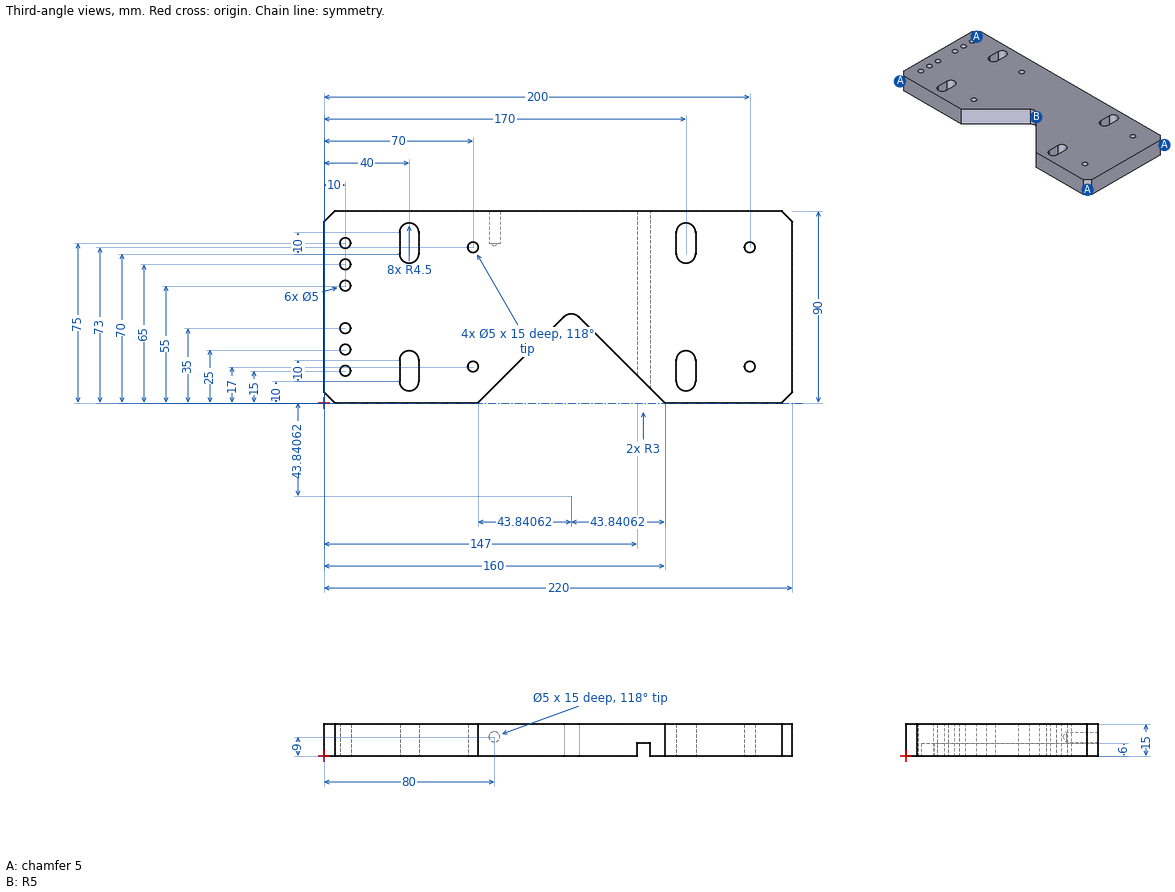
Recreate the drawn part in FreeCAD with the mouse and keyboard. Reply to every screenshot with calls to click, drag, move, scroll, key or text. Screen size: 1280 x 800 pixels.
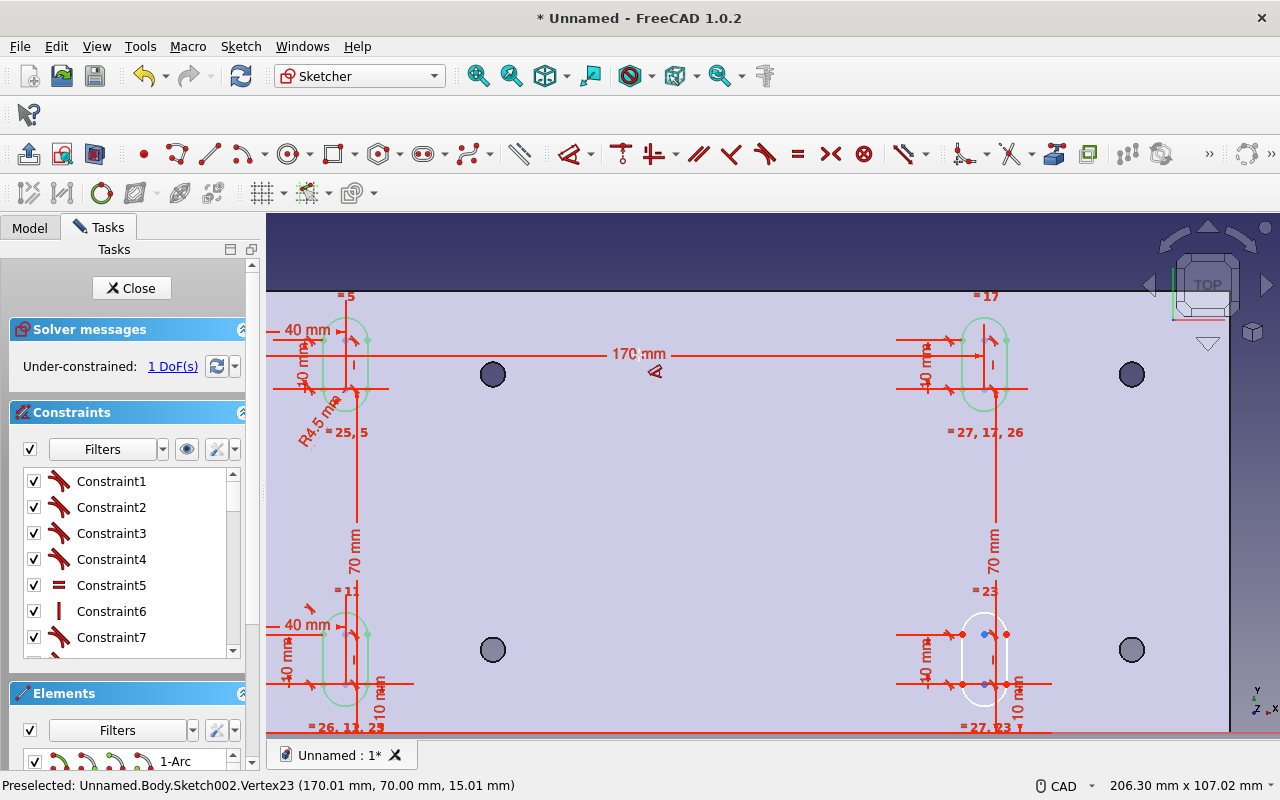
click(985, 684)
click(639, 650)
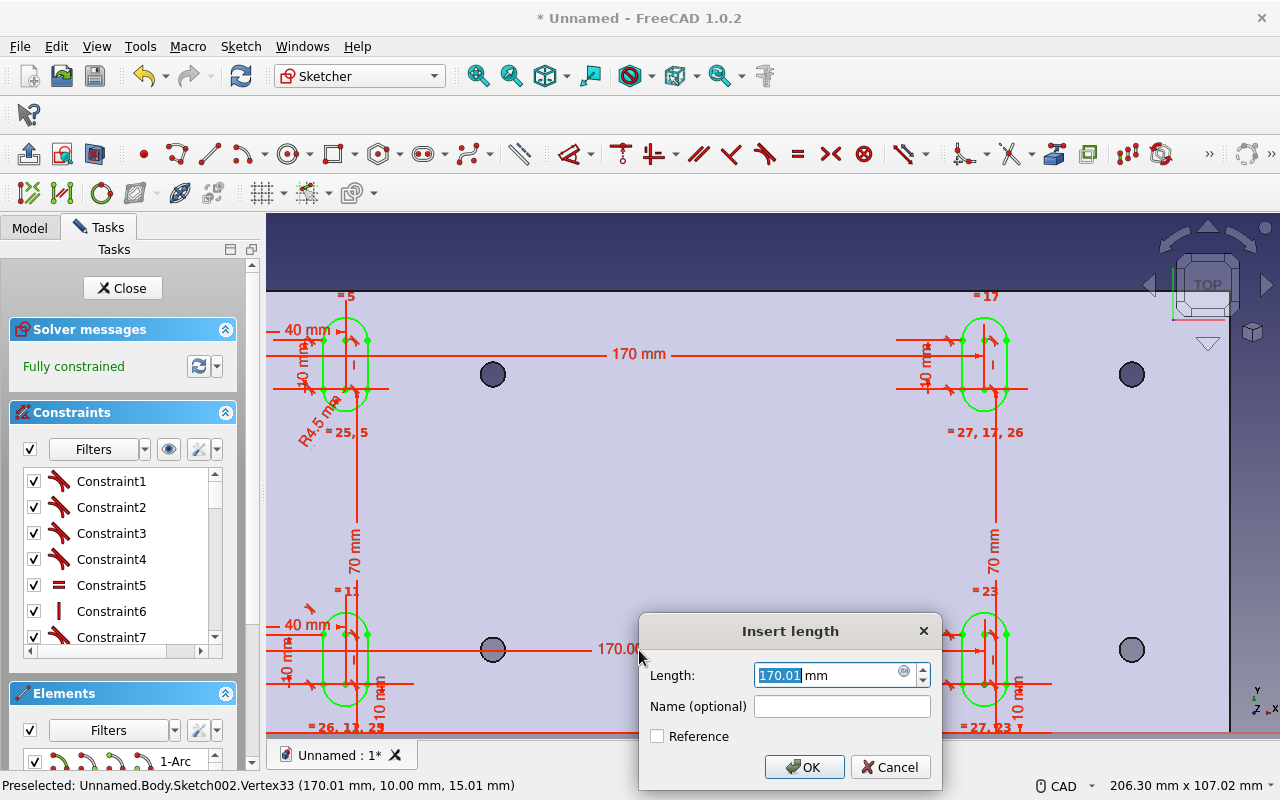
text(170)
key(Return)
key(Escape)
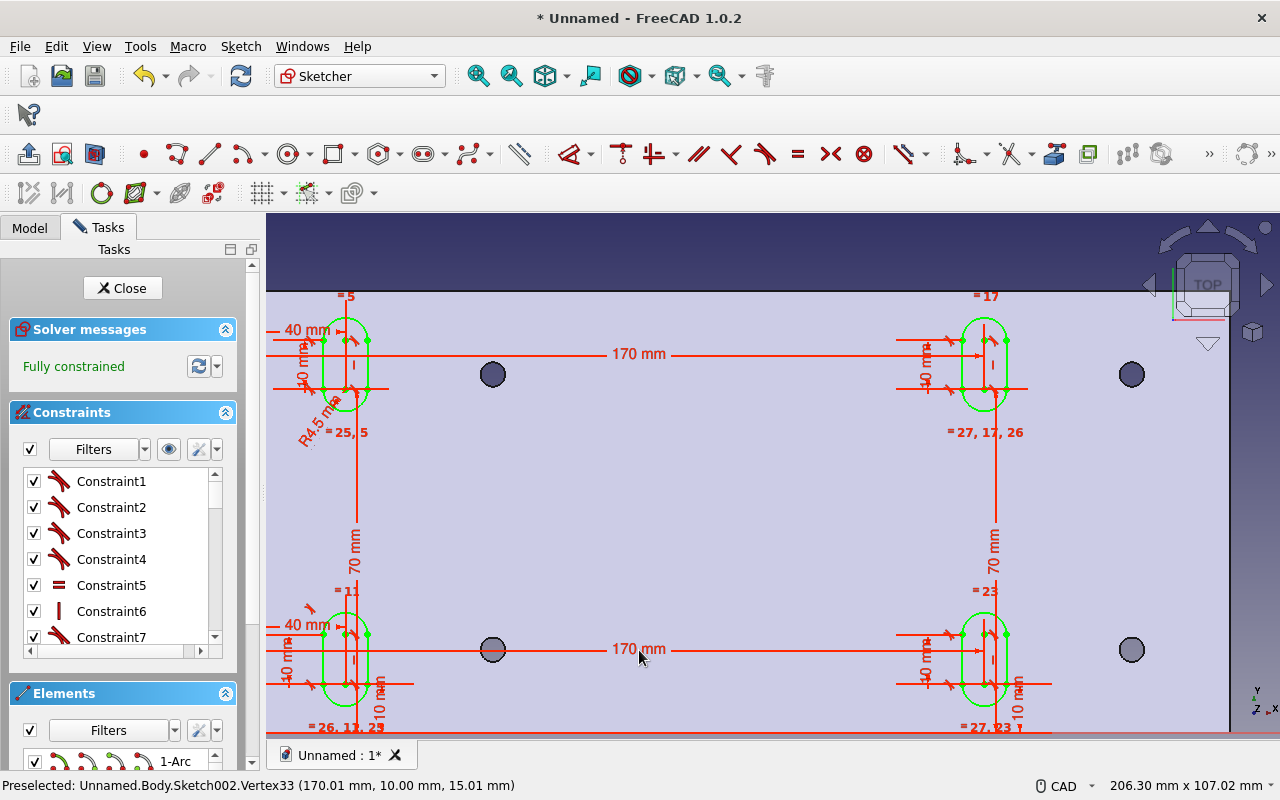
click(123, 288)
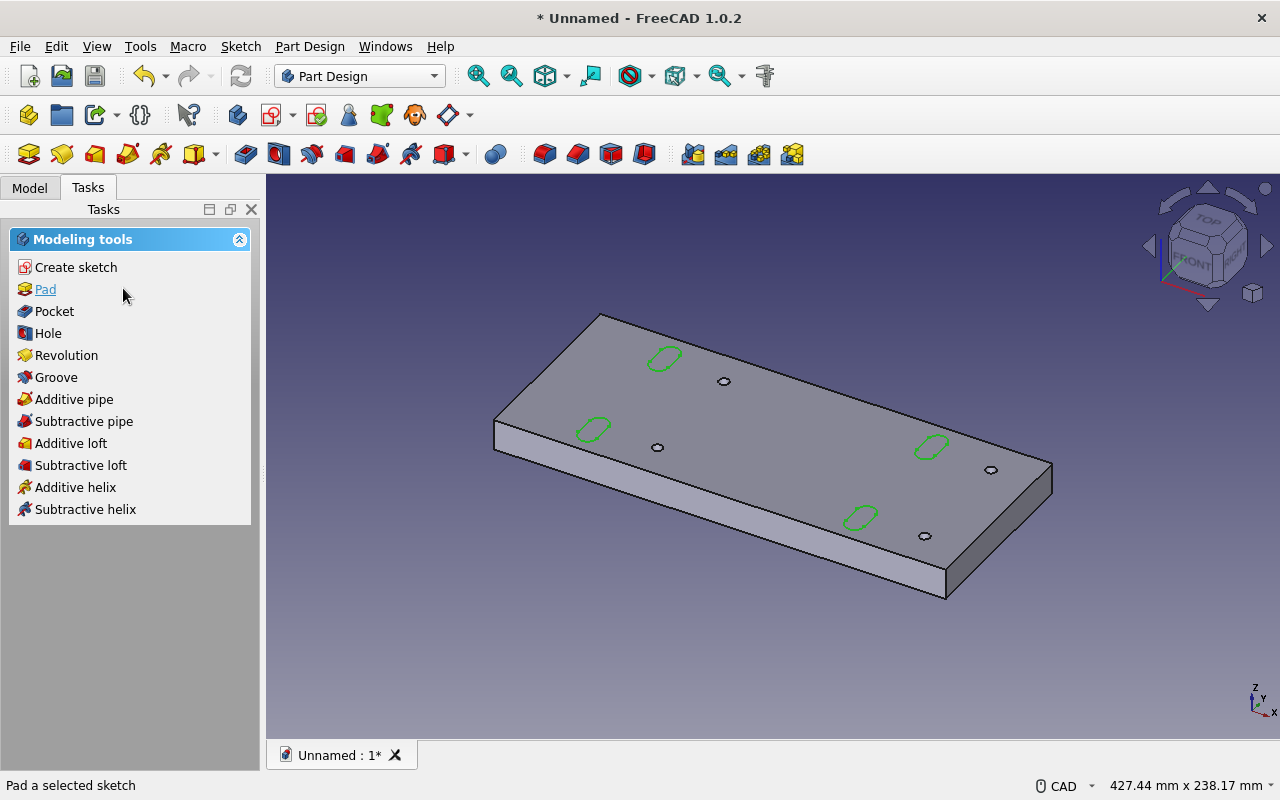
click(246, 154)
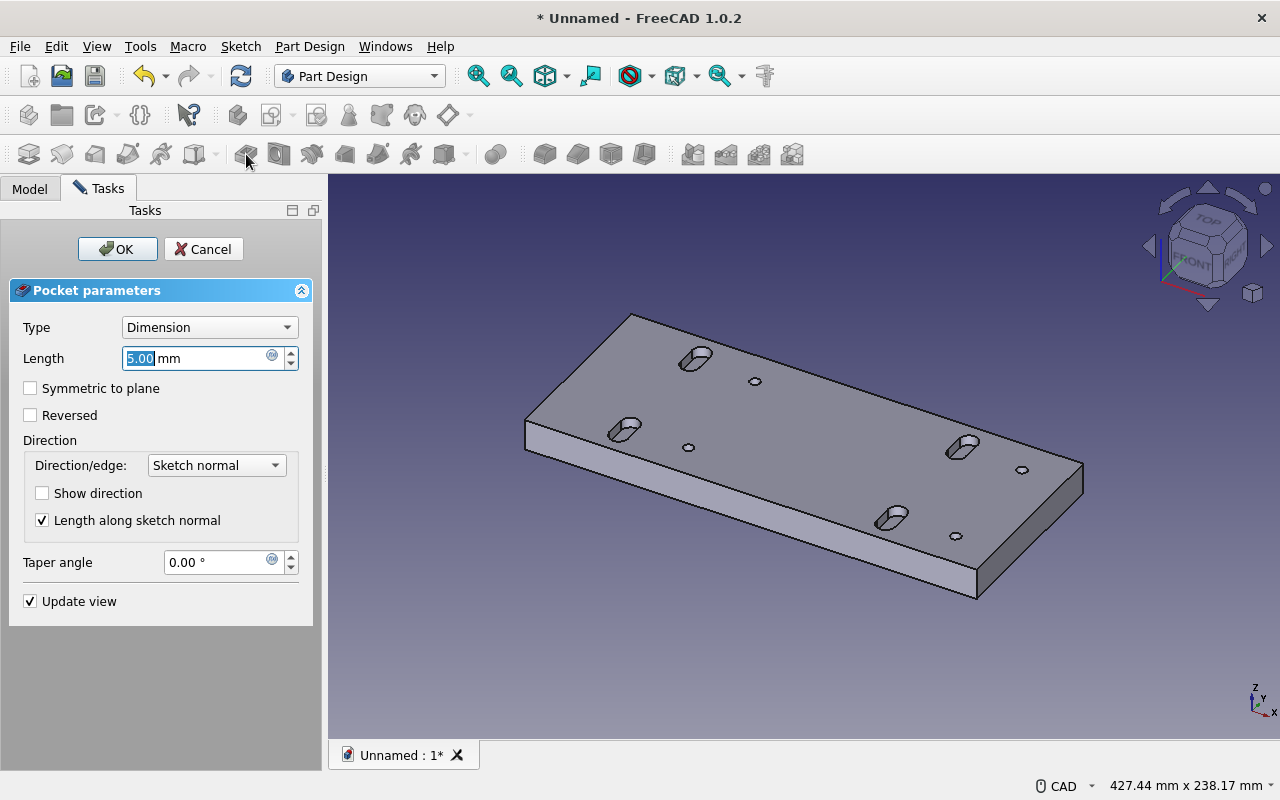
click(210, 328)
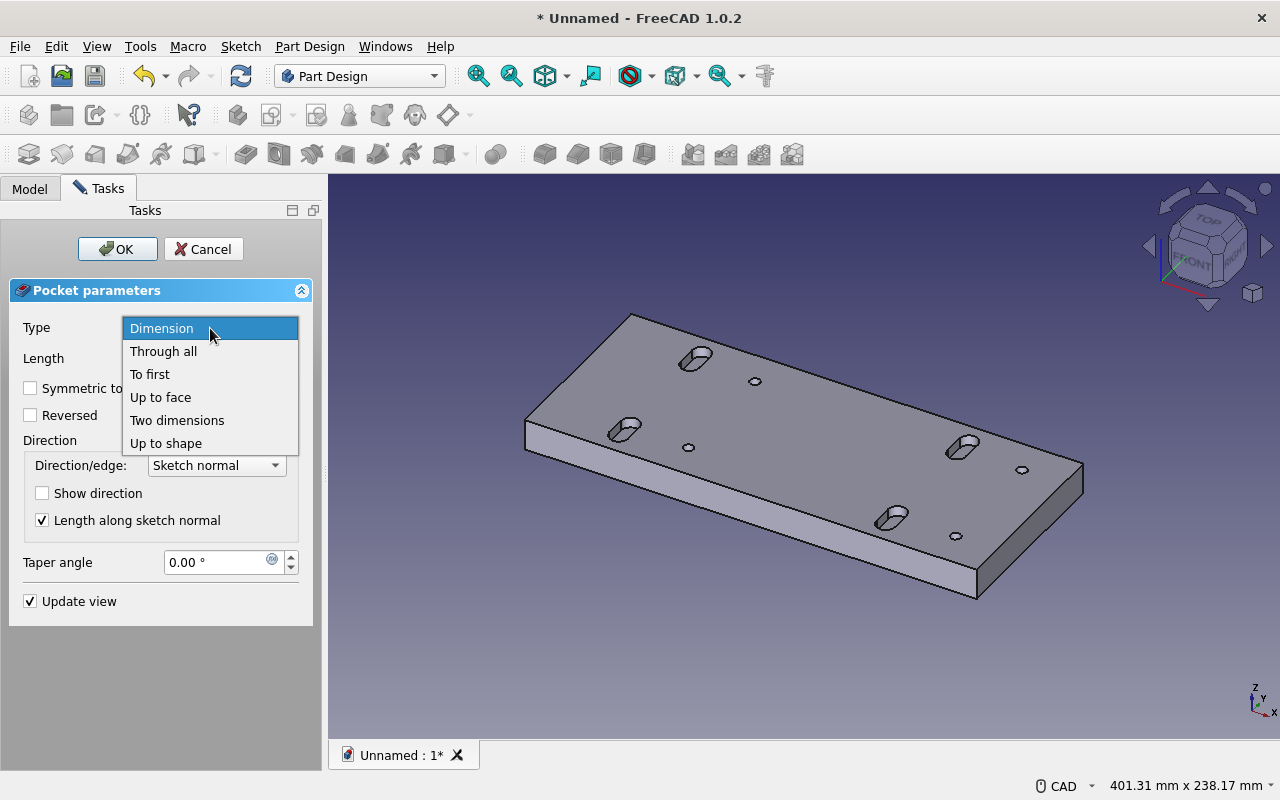
click(208, 352)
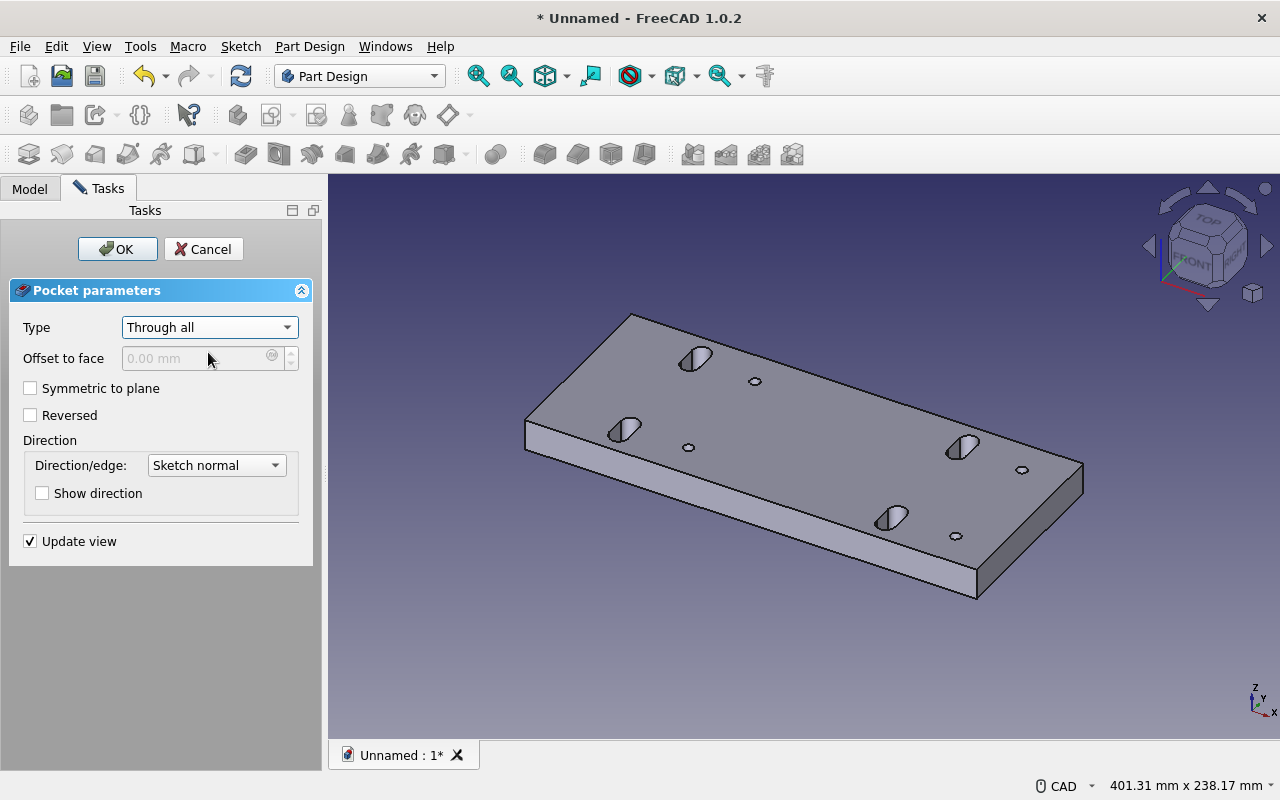
click(118, 249)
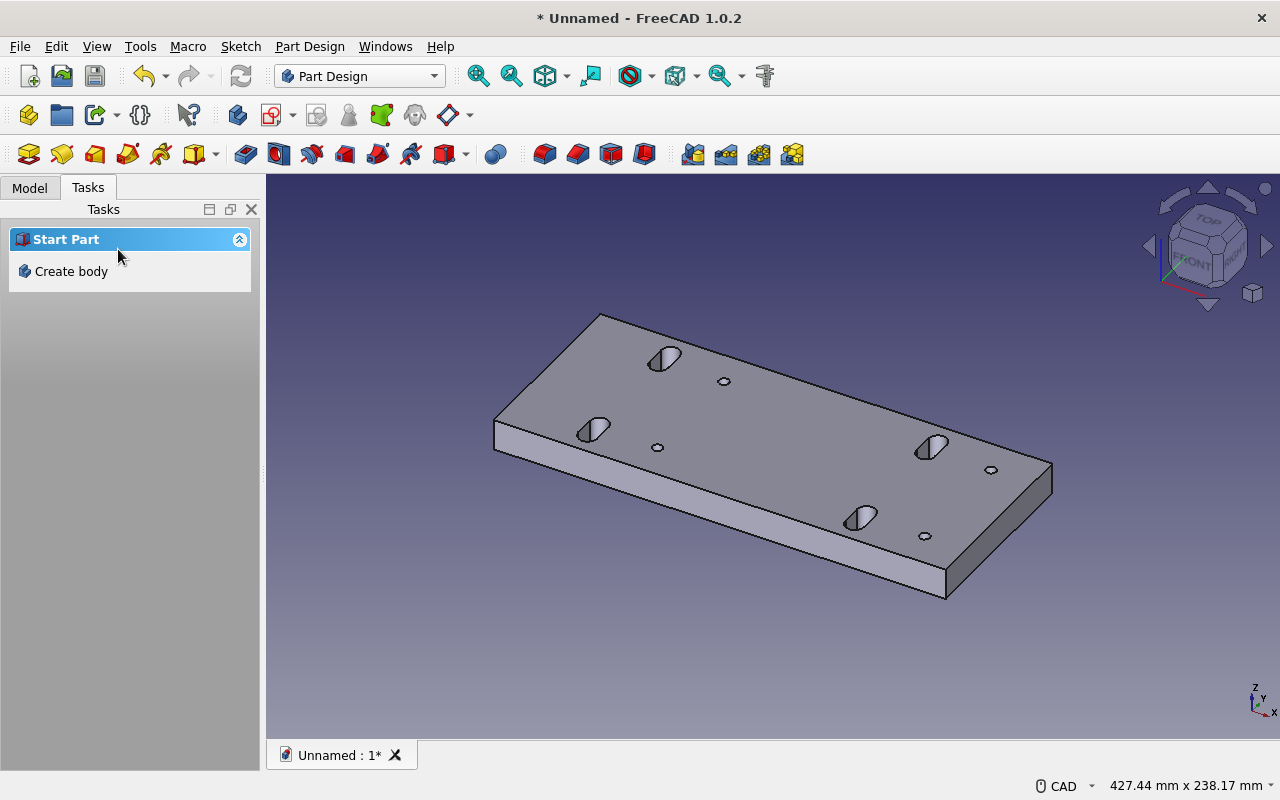
click(773, 441)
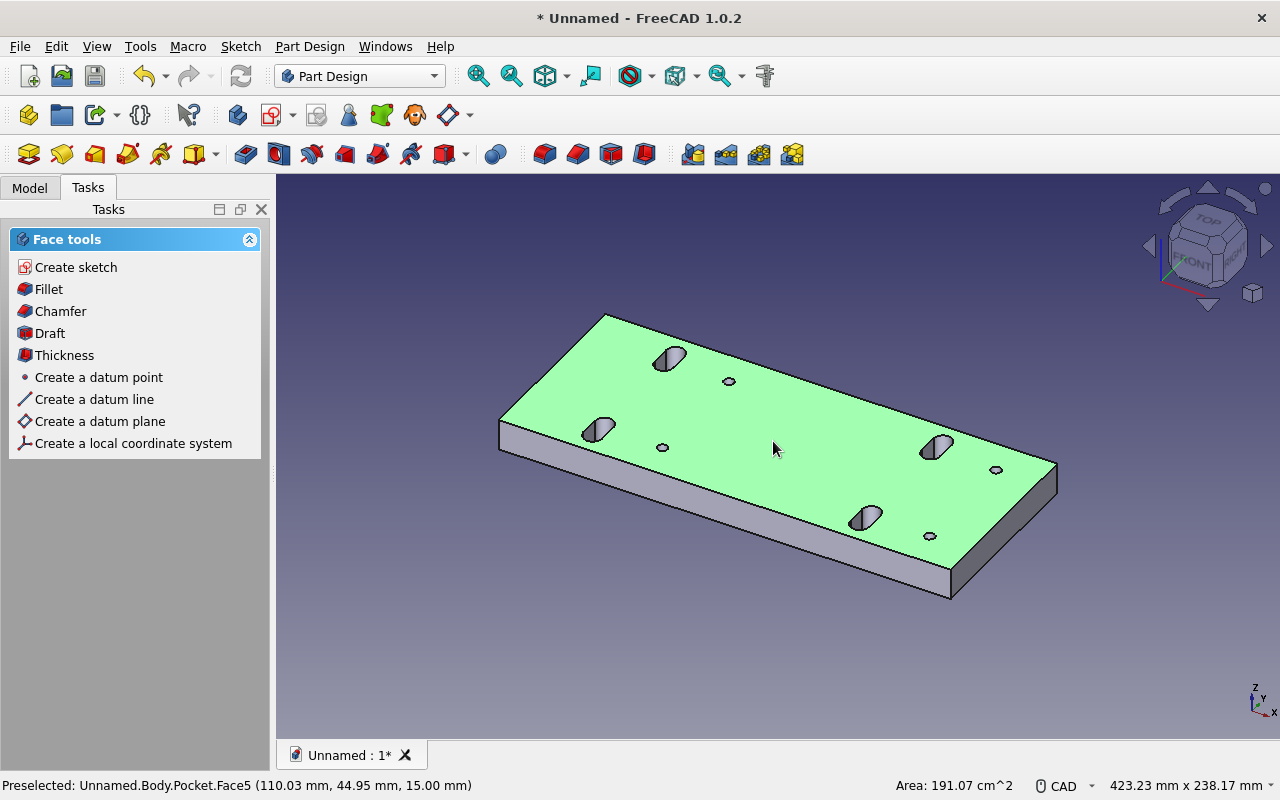
click(270, 116)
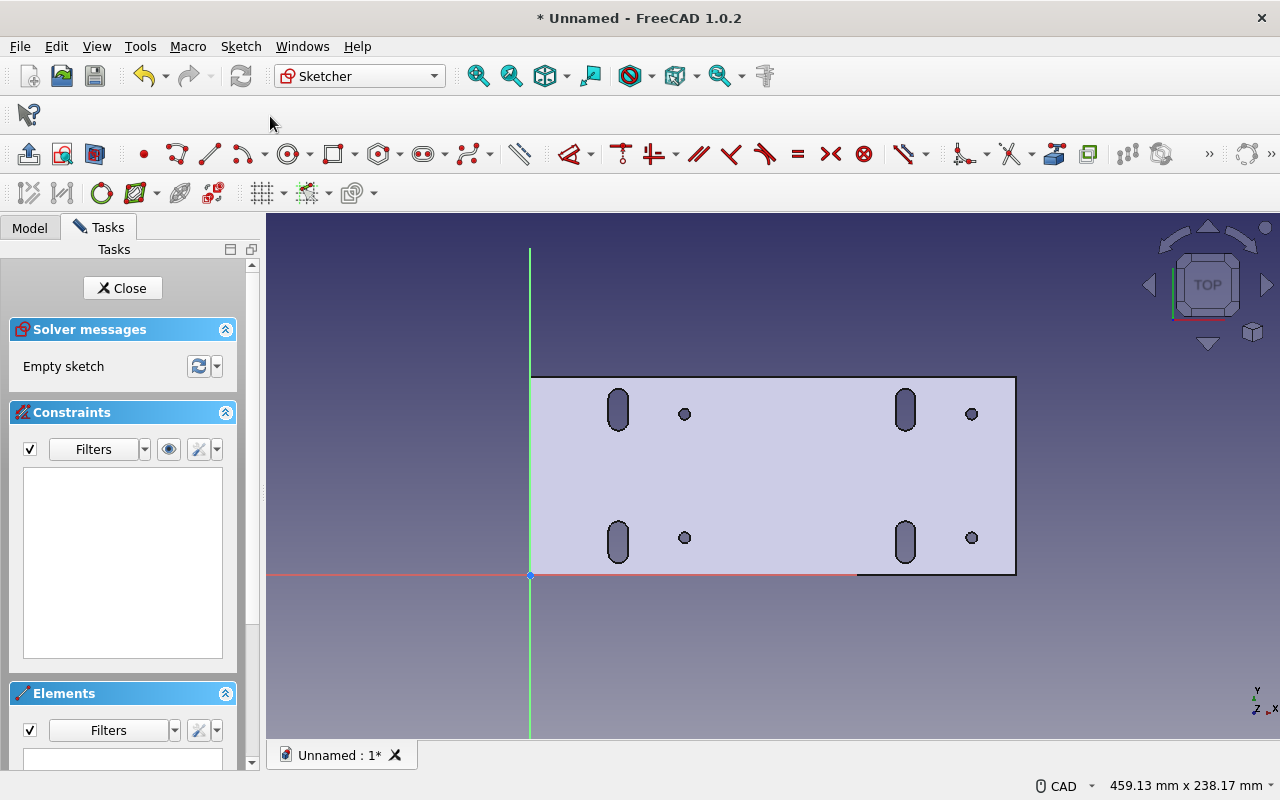
scroll(711, 711, up, 2)